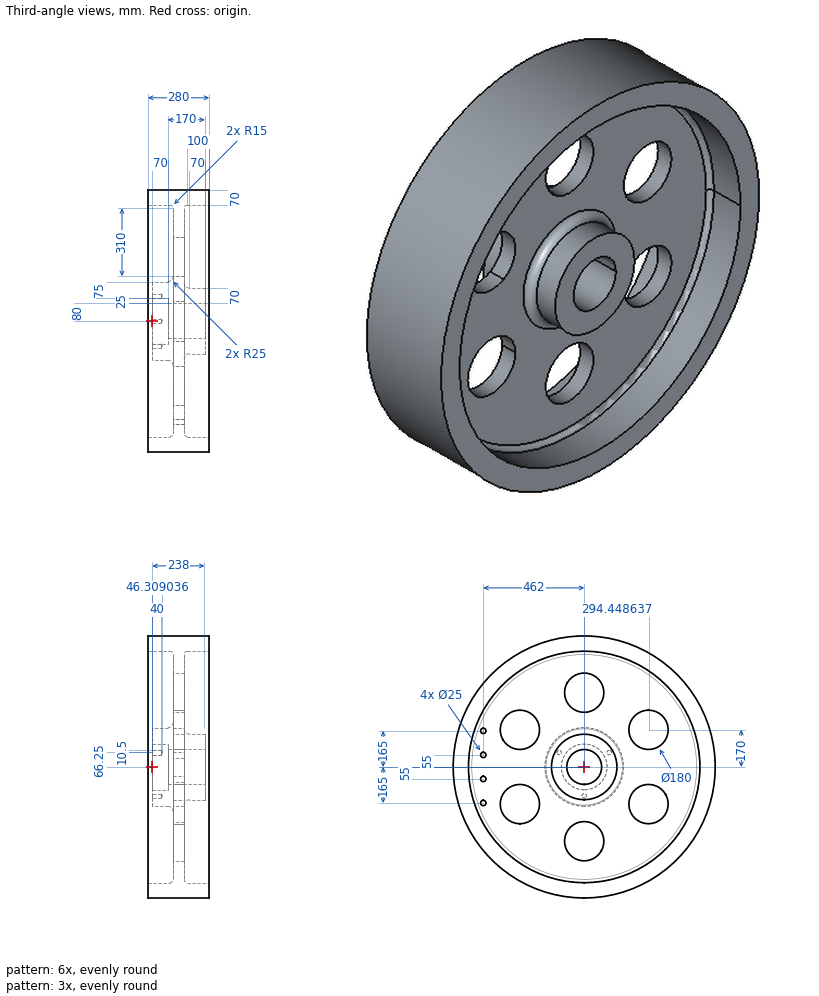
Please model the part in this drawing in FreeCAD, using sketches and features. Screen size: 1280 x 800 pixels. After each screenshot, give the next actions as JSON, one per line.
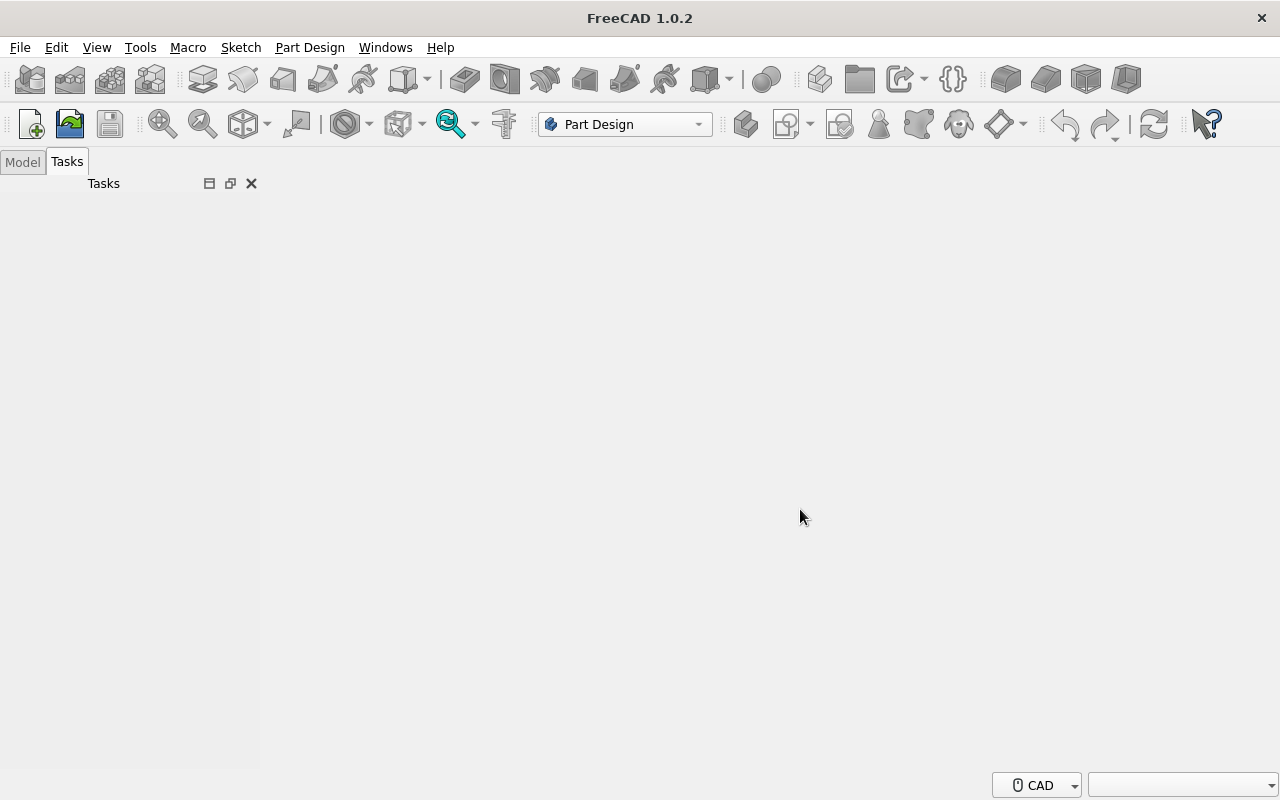
{"action": "key", "text": "ctrl+n"}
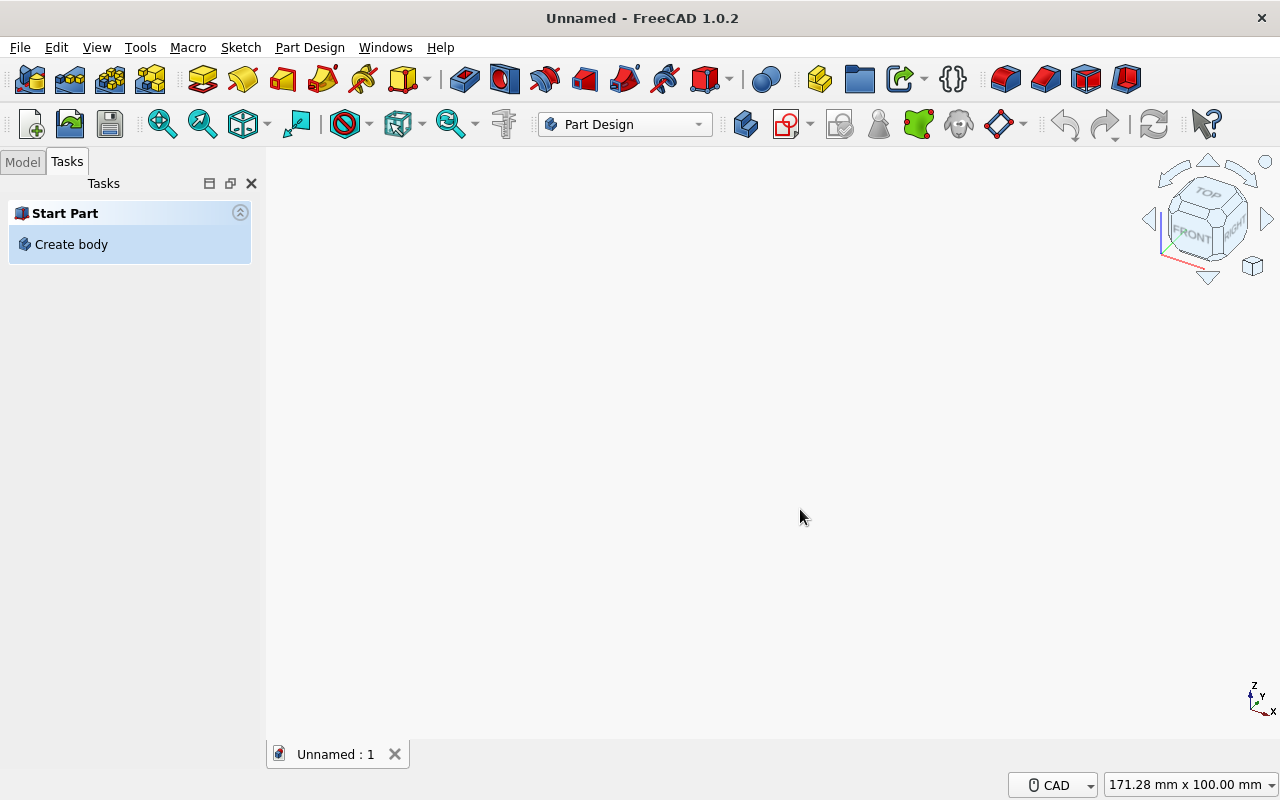
{"action": "left_click", "coordinate": [786, 124]}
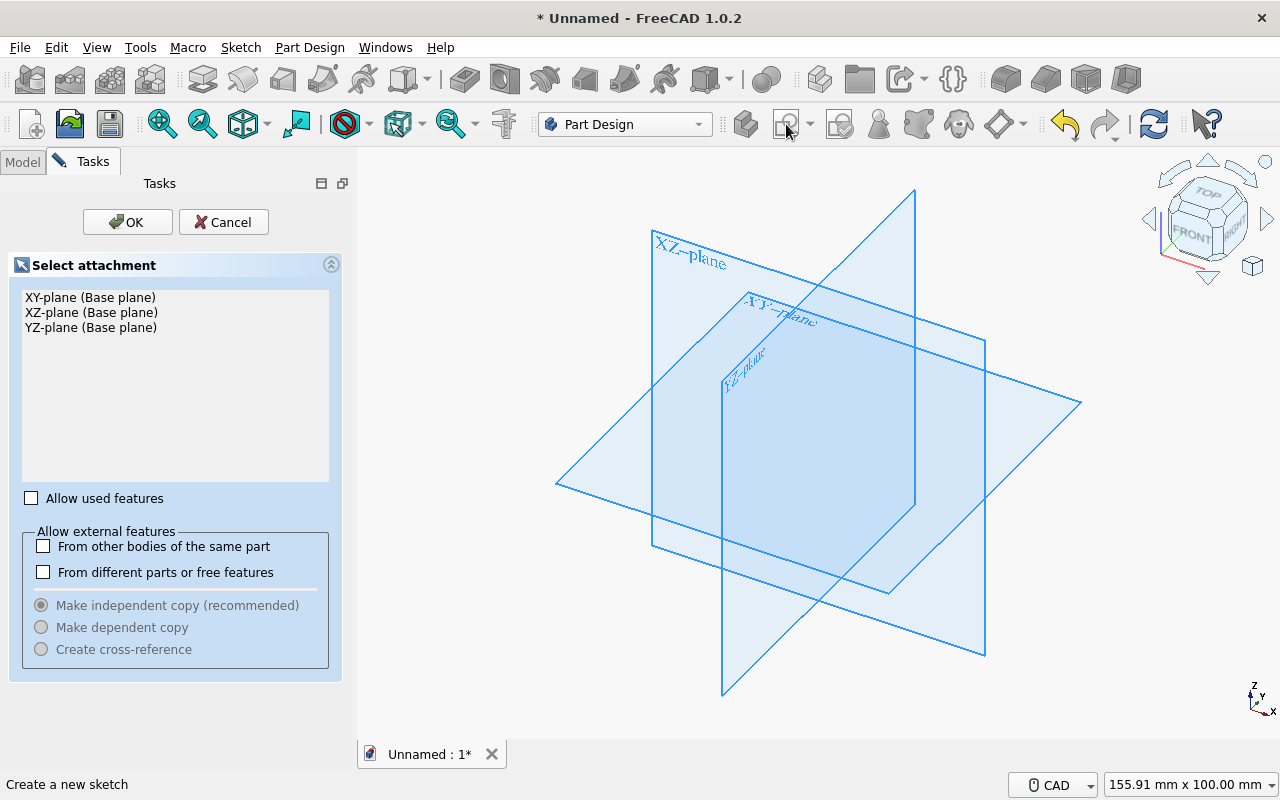
{"action": "left_click", "coordinate": [82, 298]}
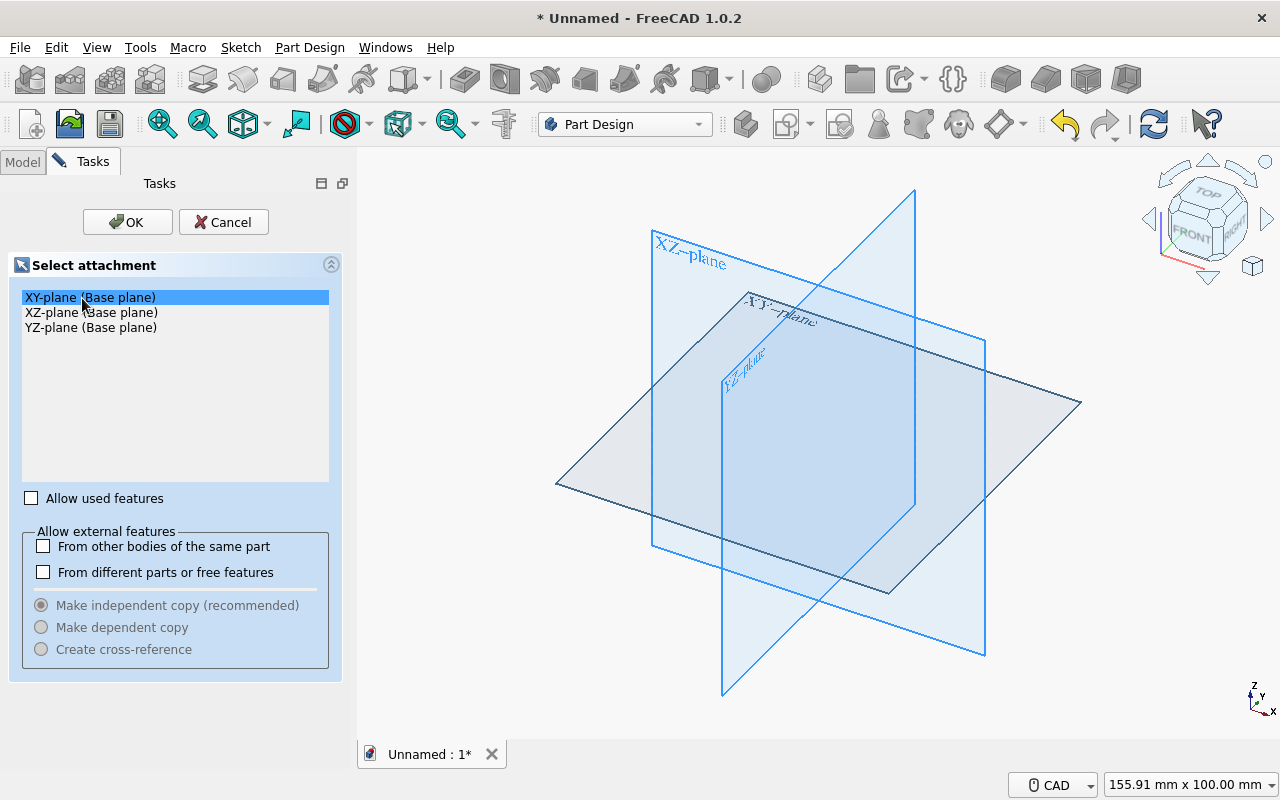
{"action": "left_click", "coordinate": [128, 222]}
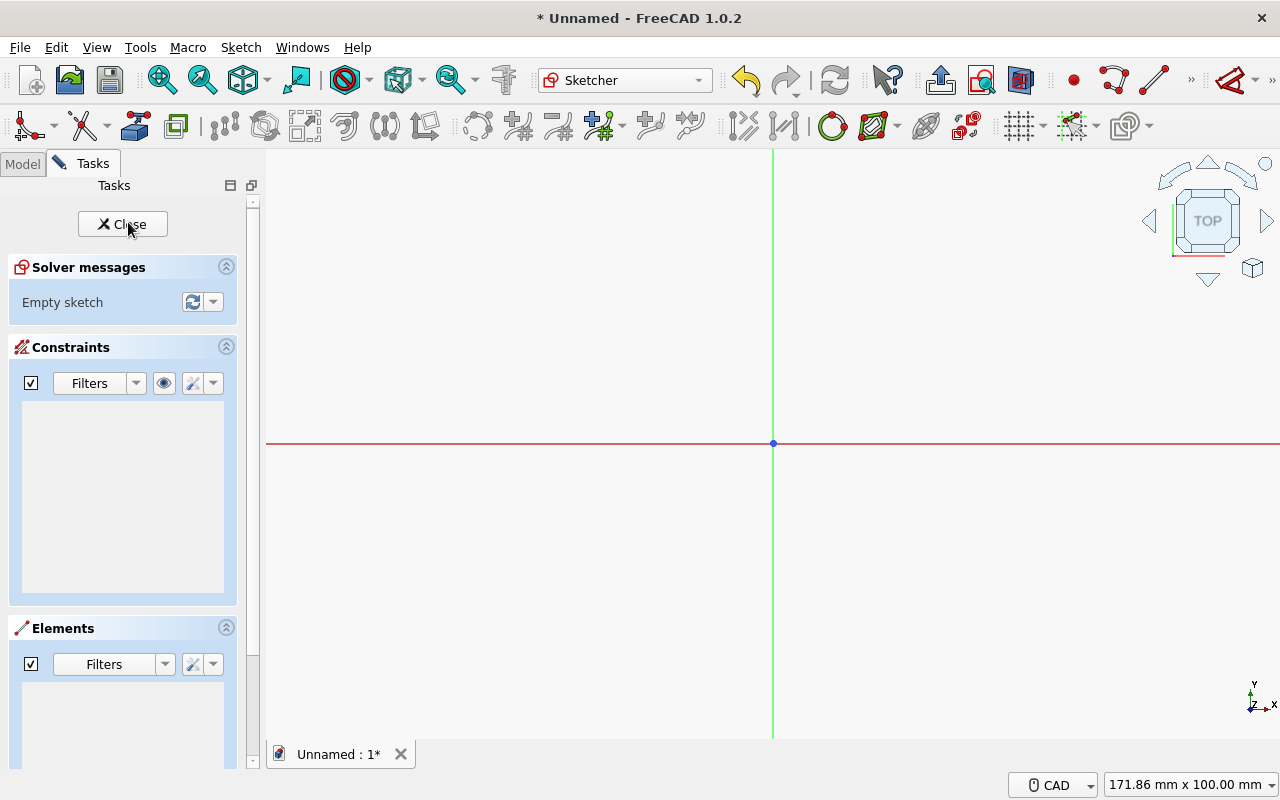
{"action": "scroll", "coordinate": [608, 665], "scroll_direction": "down", "scroll_amount": 11}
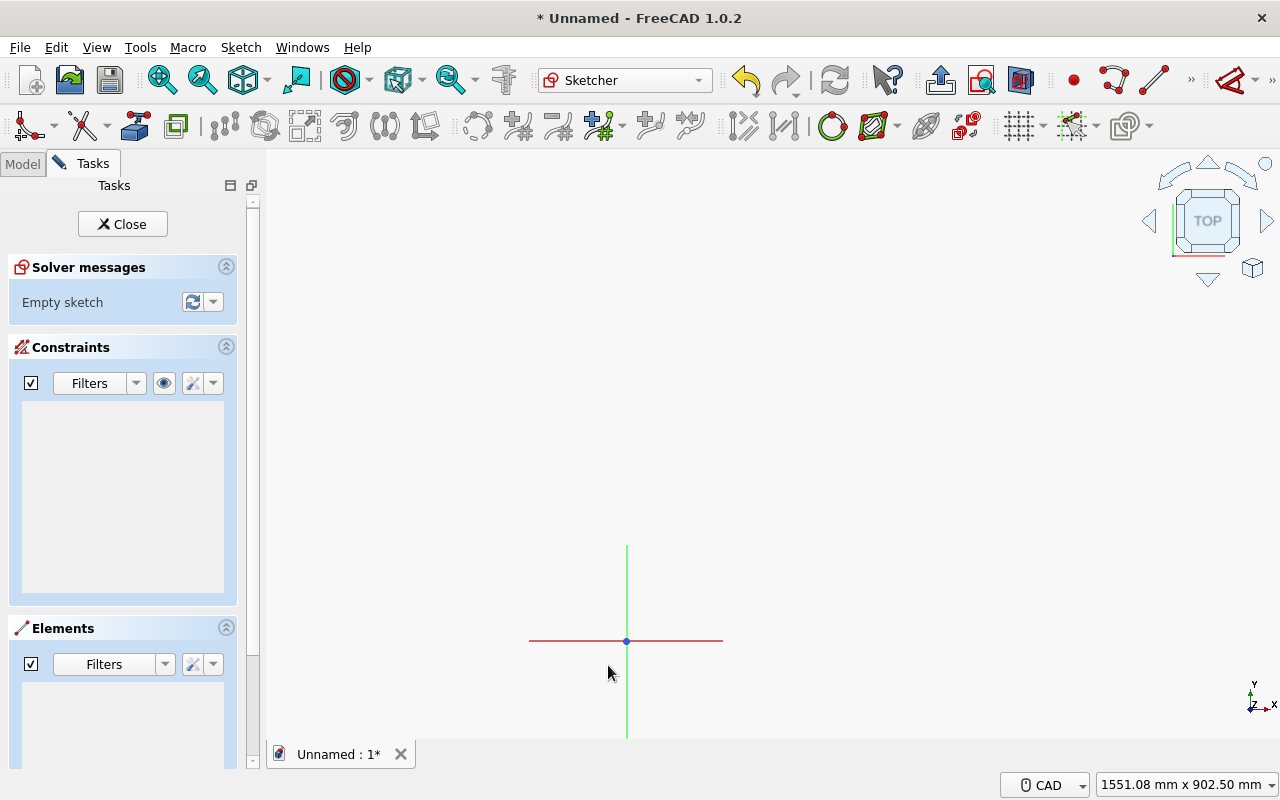
{"action": "key", "text": "g l"}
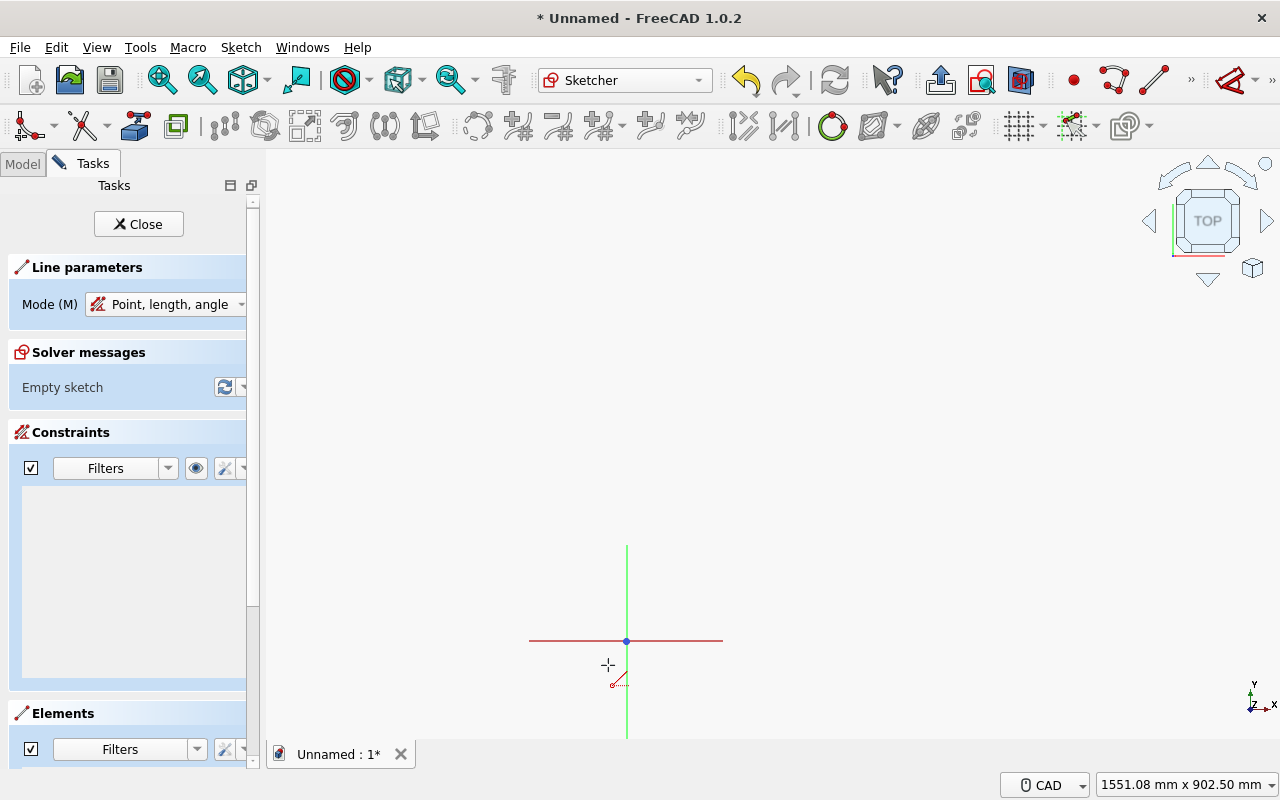
{"action": "left_click", "coordinate": [689, 305]}
{"action": "left_click", "coordinate": [689, 507]}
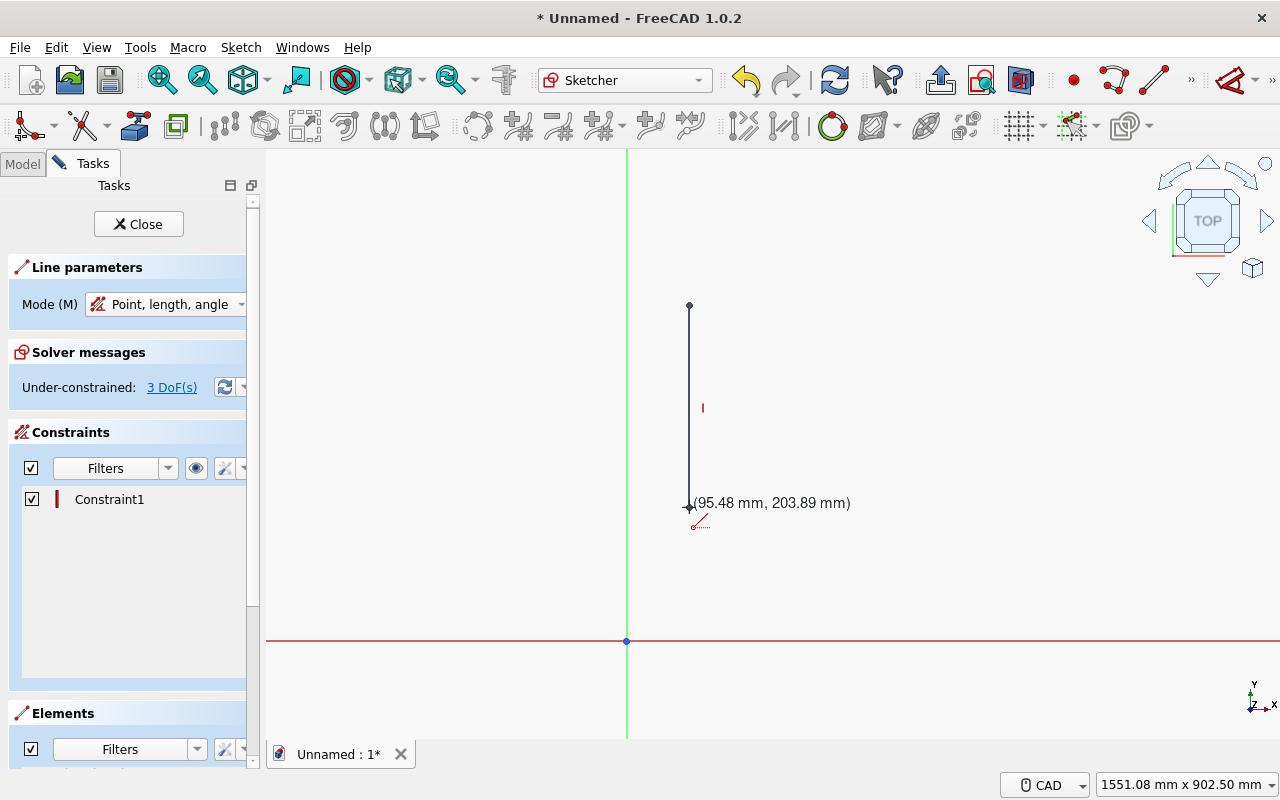
{"action": "left_click", "coordinate": [1114, 80]}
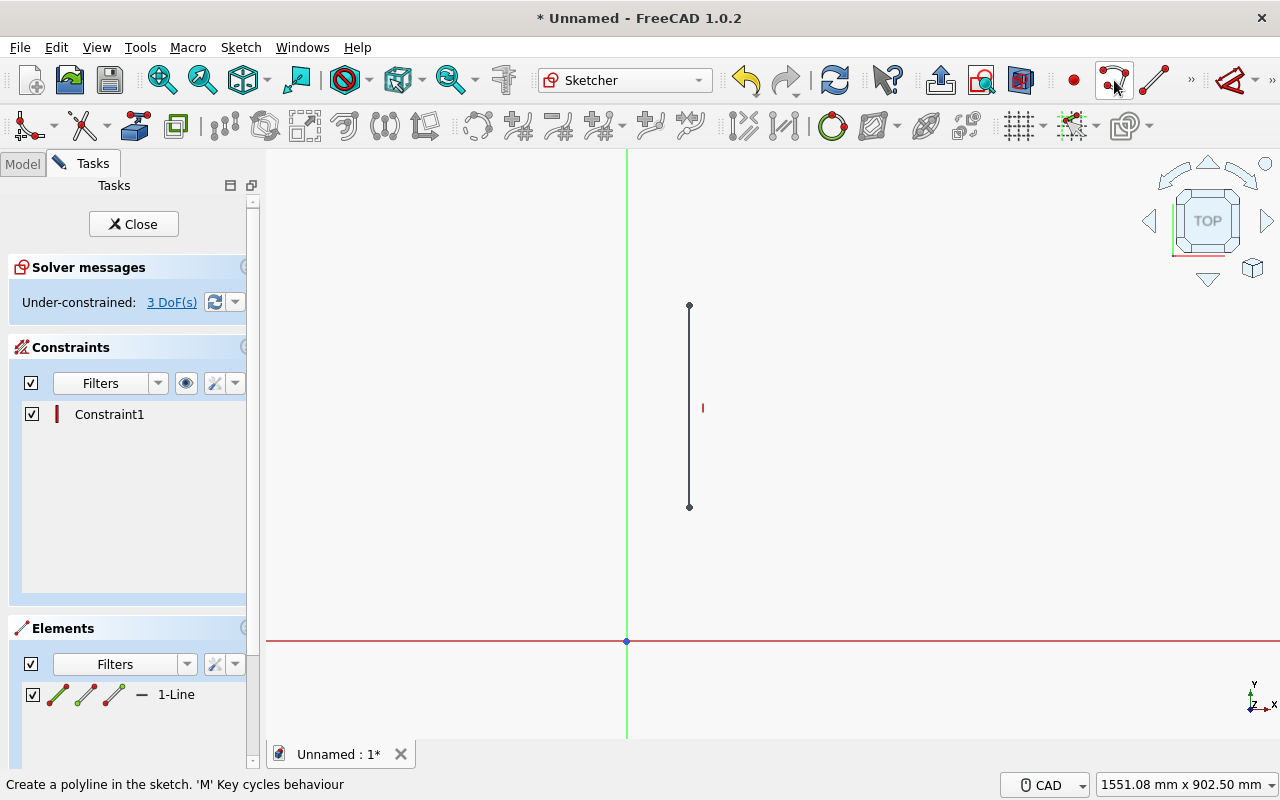
{"action": "left_click", "coordinate": [672, 524]}
{"action": "left_click", "coordinate": [627, 524]}
{"action": "left_click", "coordinate": [636, 573]}
{"action": "left_click", "coordinate": [672, 573]}
{"action": "left_click", "coordinate": [672, 589]}
{"action": "left_click", "coordinate": [783, 589]}
{"action": "left_click", "coordinate": [783, 543]}
{"action": "left_click", "coordinate": [738, 543]}
{"action": "right_click", "coordinate": [738, 543]}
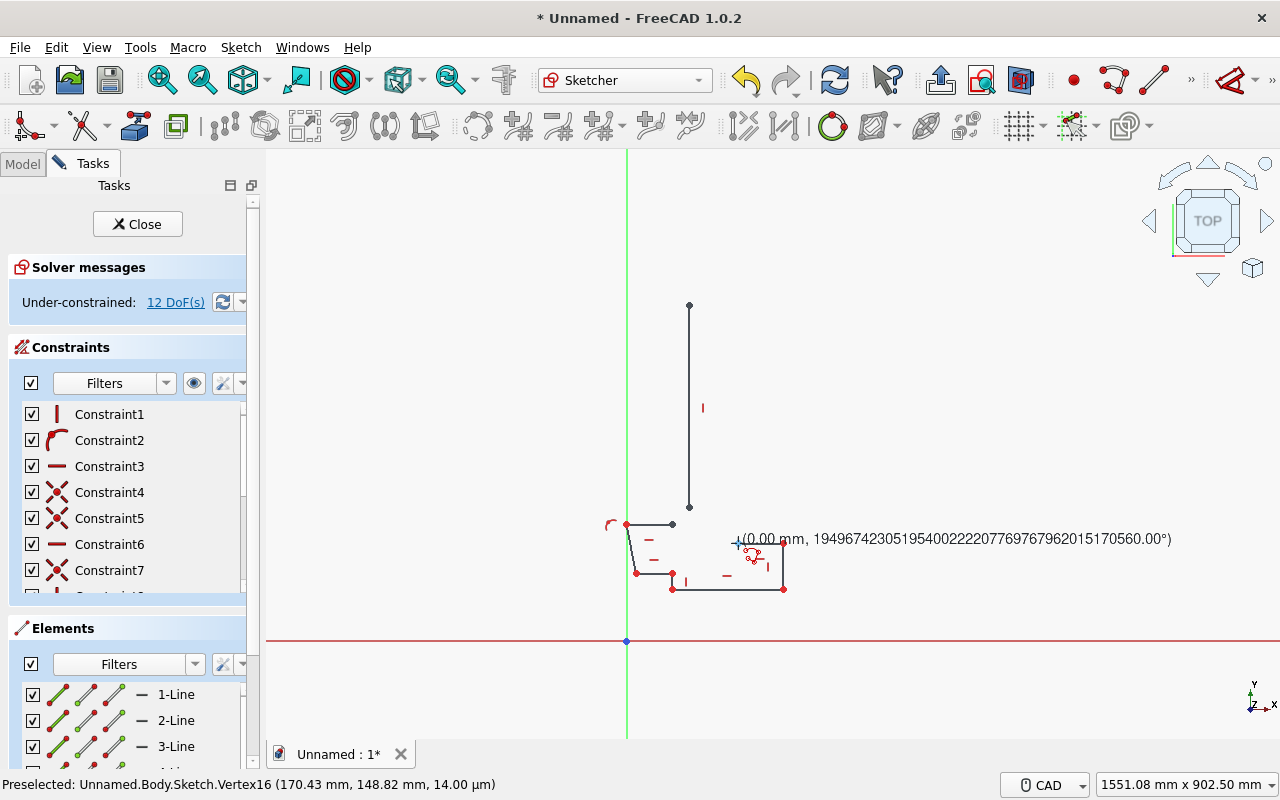
{"action": "left_click", "coordinate": [1154, 80]}